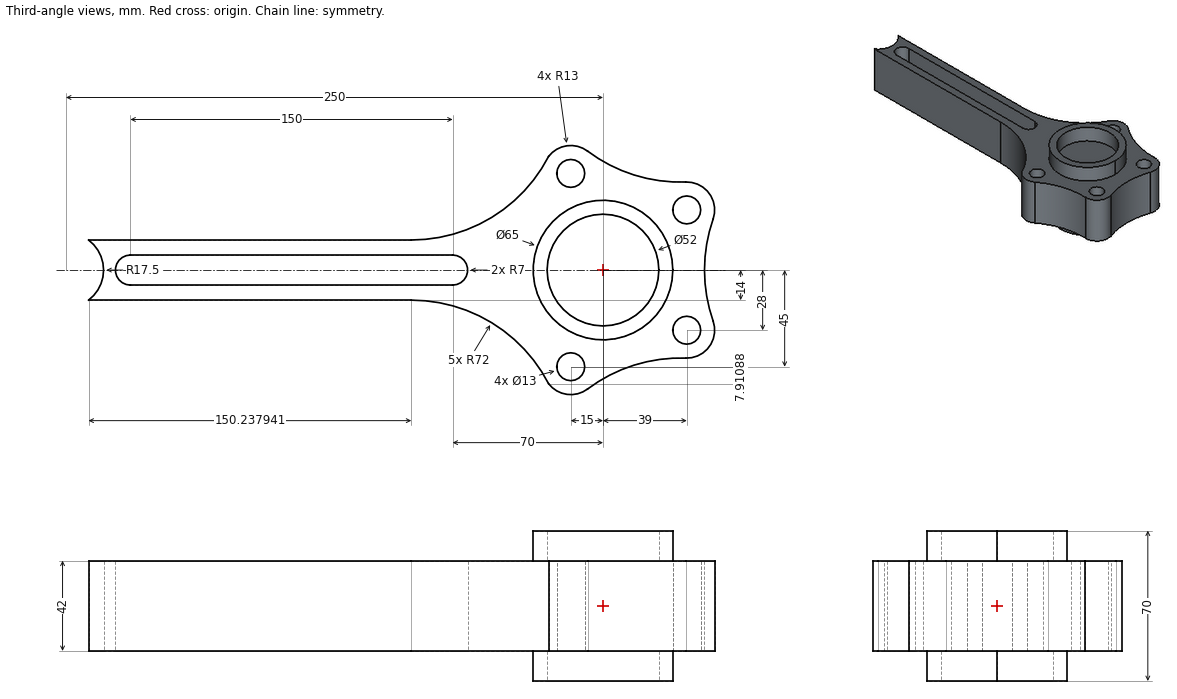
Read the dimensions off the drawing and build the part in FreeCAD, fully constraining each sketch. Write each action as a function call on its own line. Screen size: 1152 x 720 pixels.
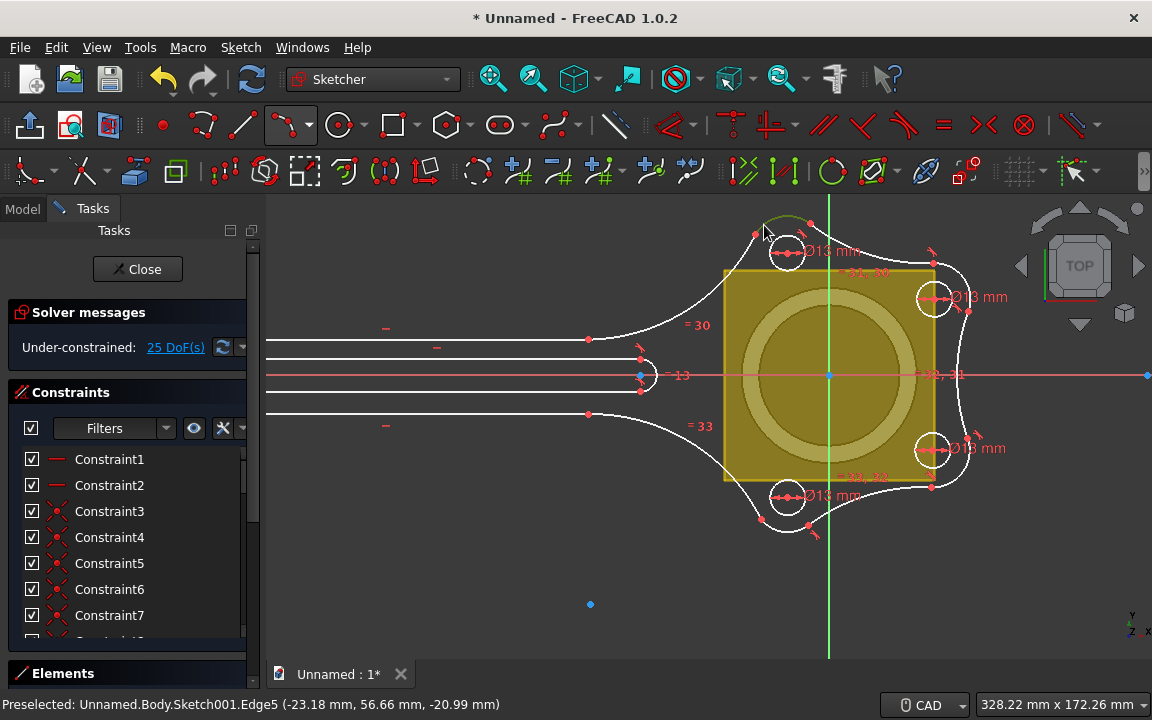
click(969, 291)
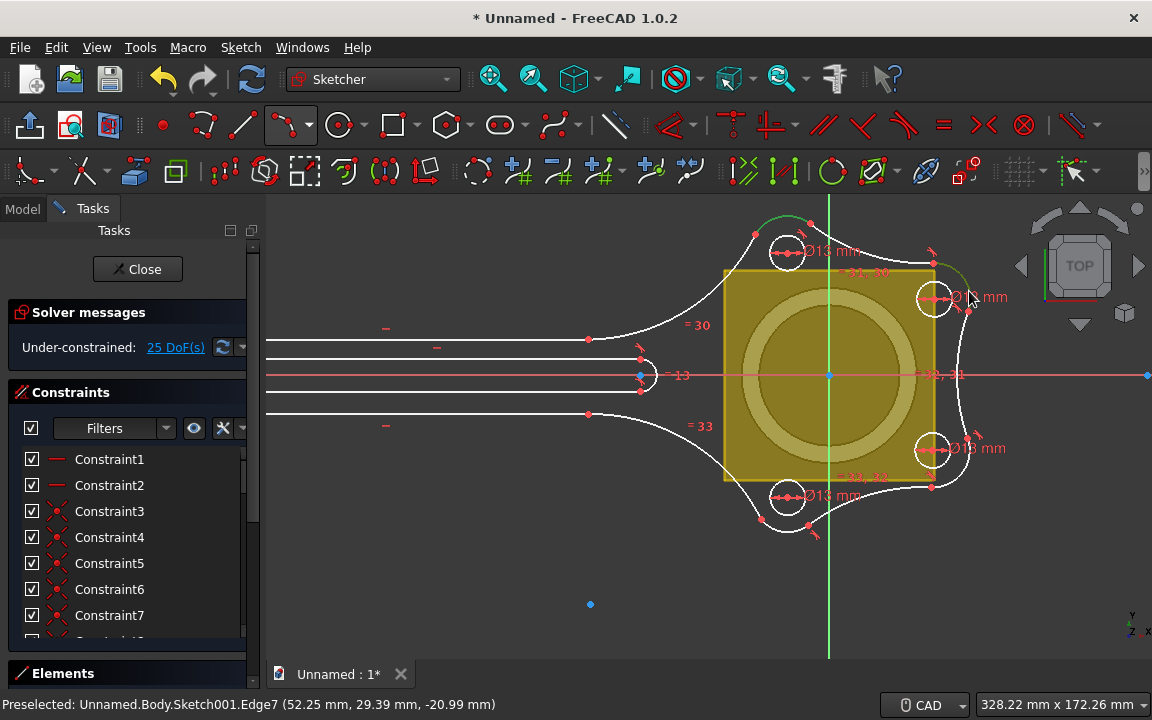
click(952, 482)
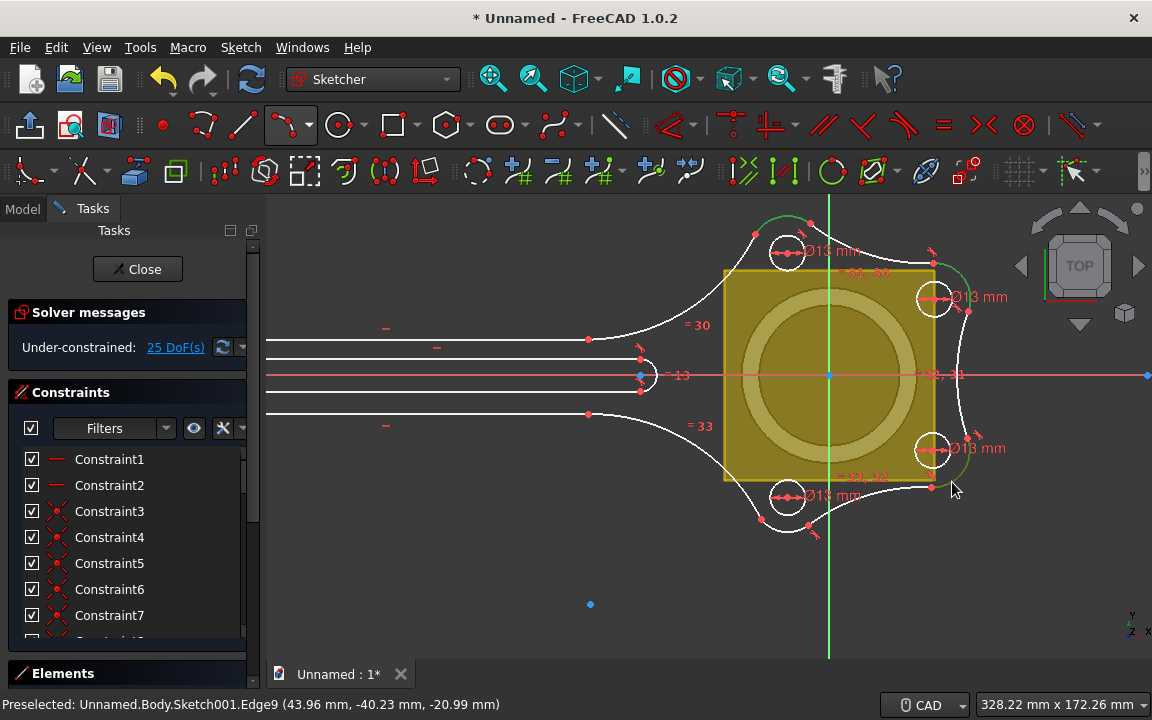
click(774, 529)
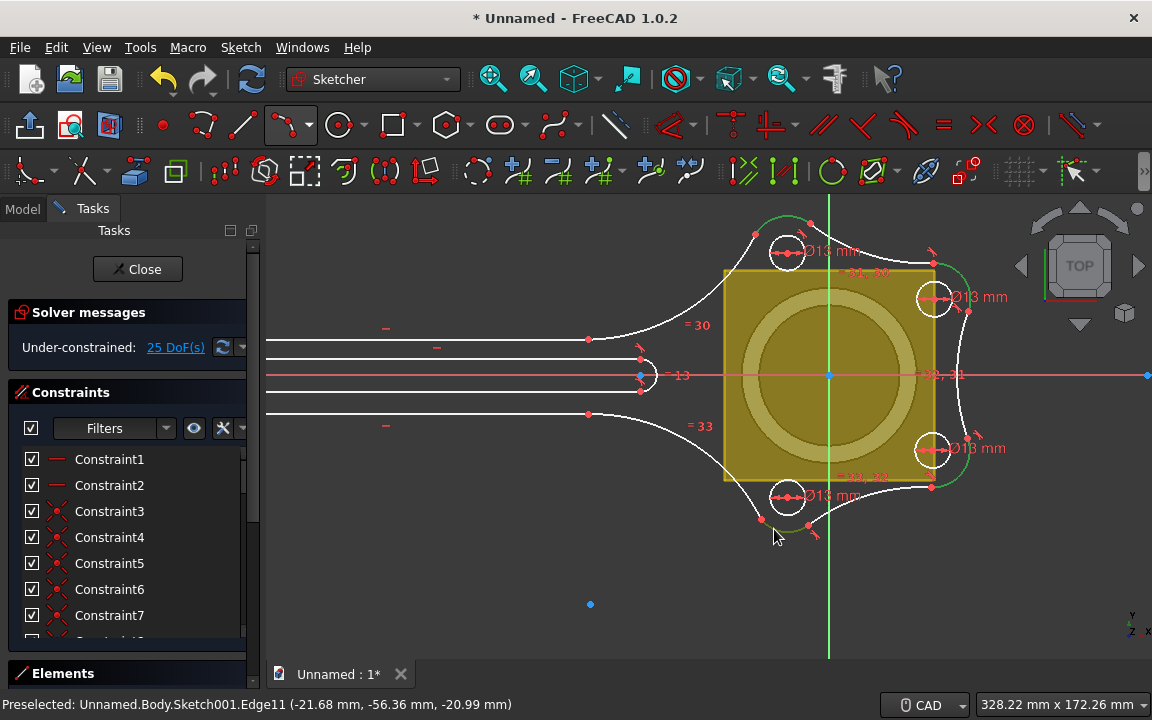
click(944, 126)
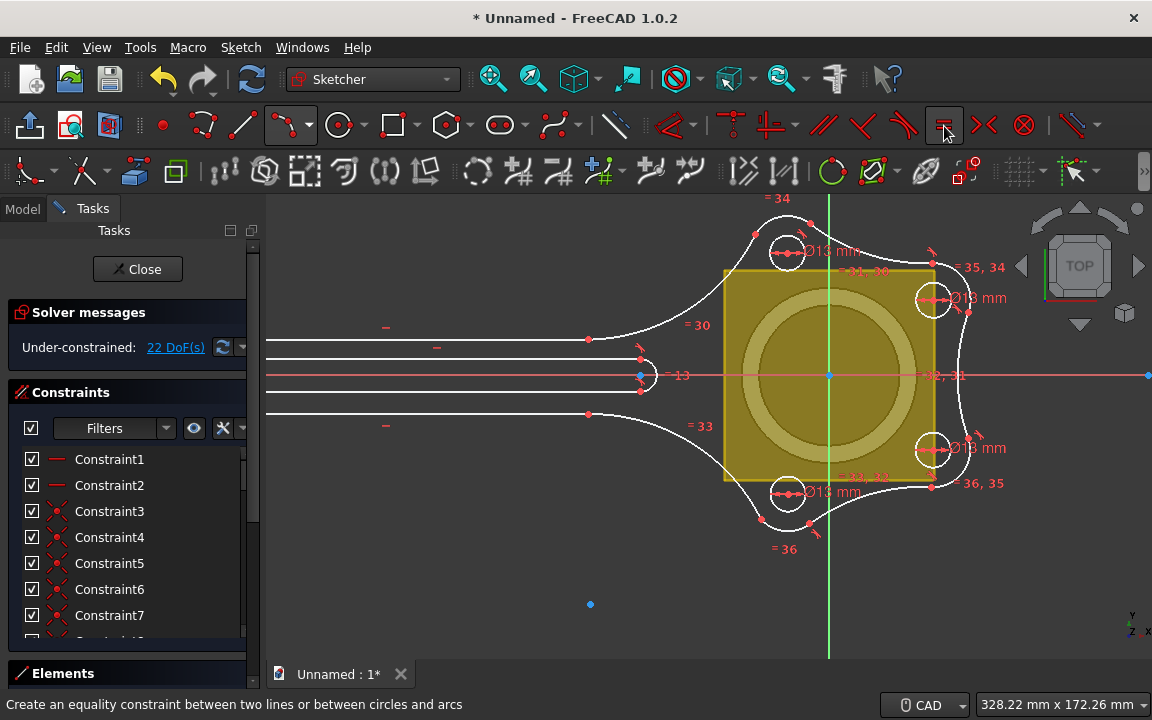
scroll(773, 530, down, 2)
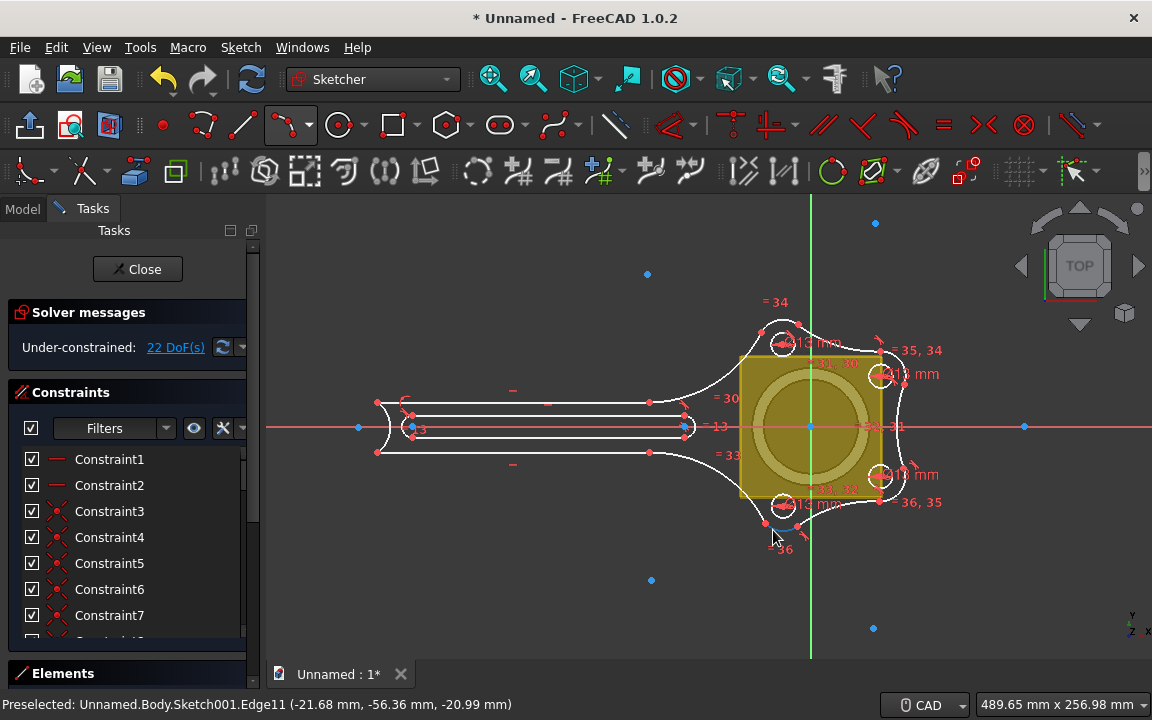
click(359, 428)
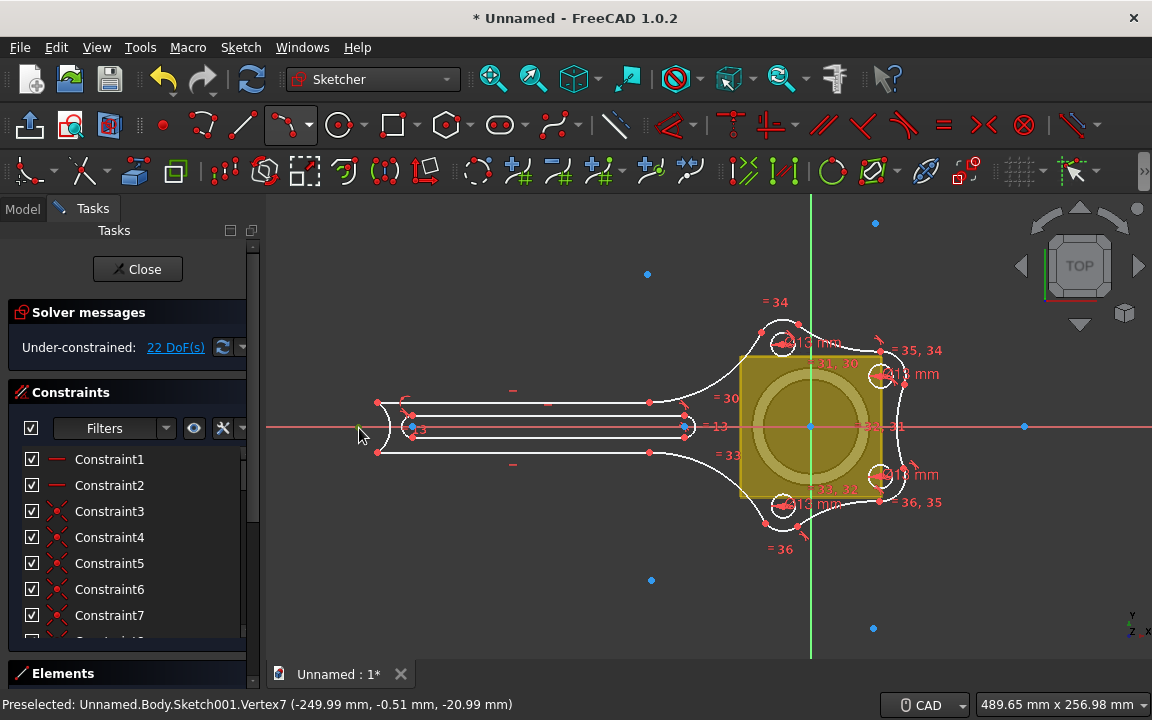
click(344, 427)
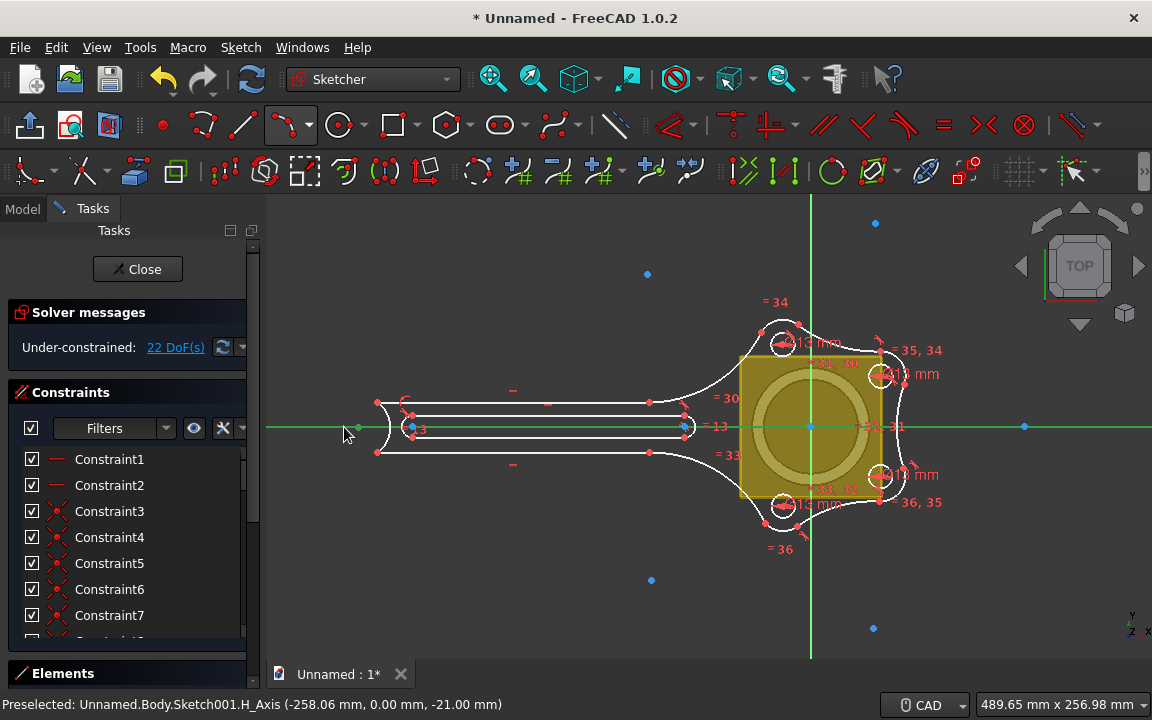
click(732, 126)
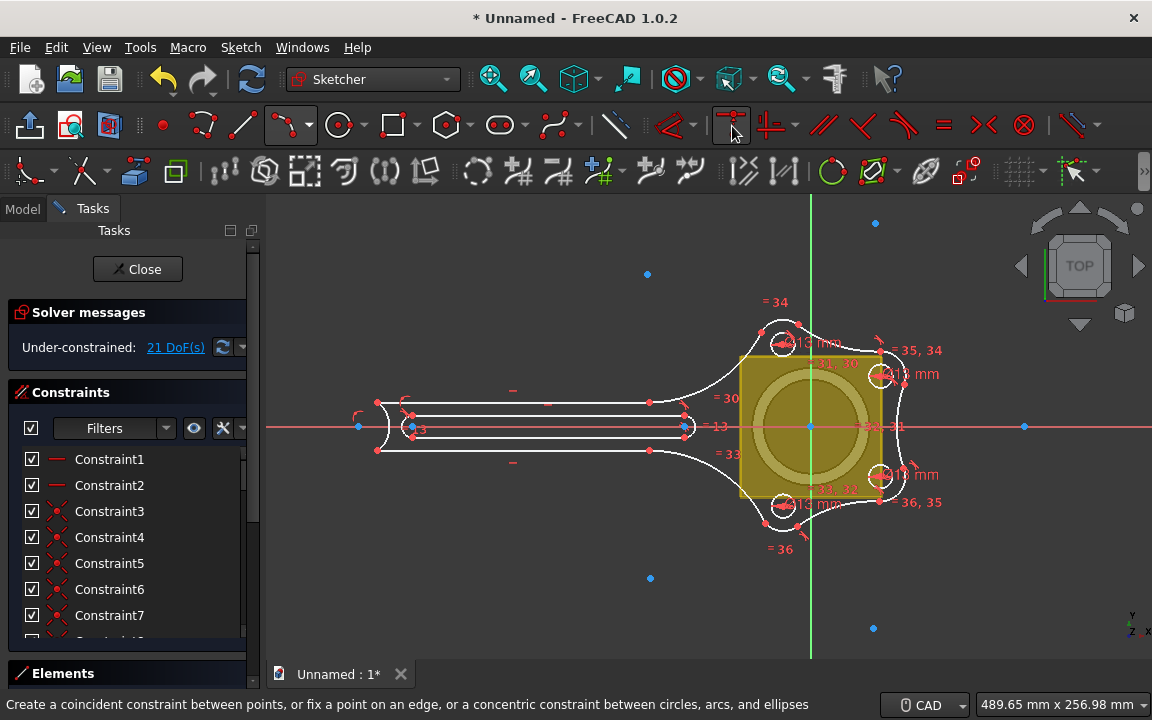
scroll(367, 426, down, 1)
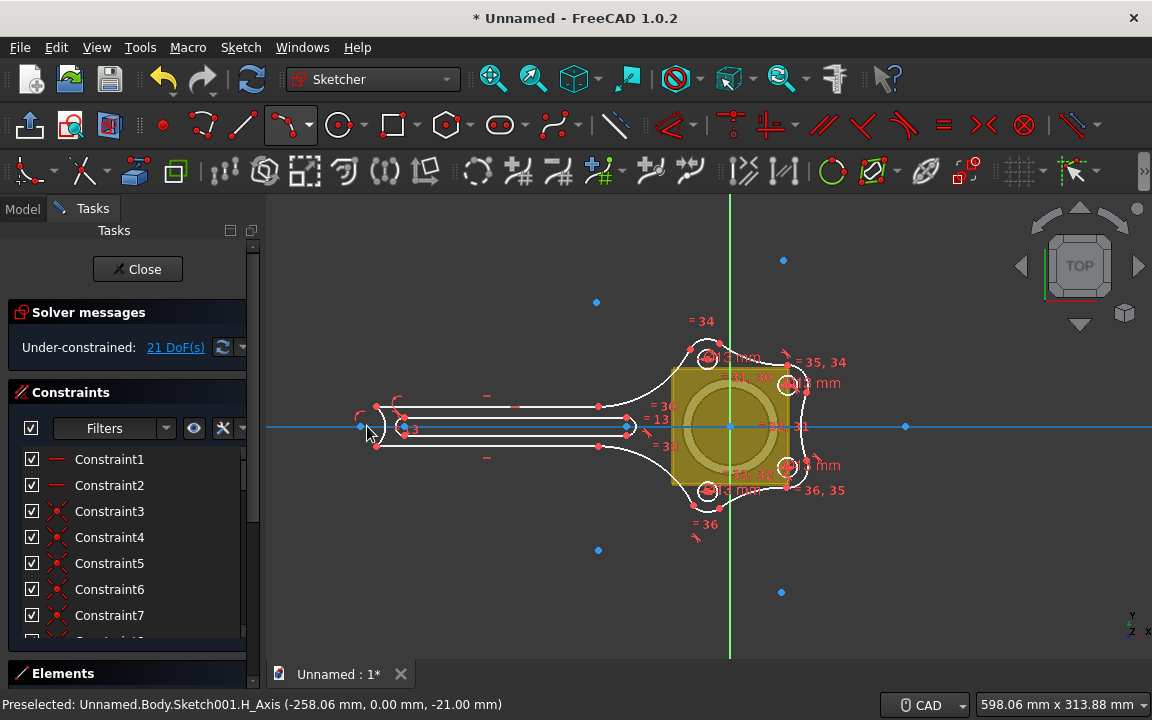
click(905, 427)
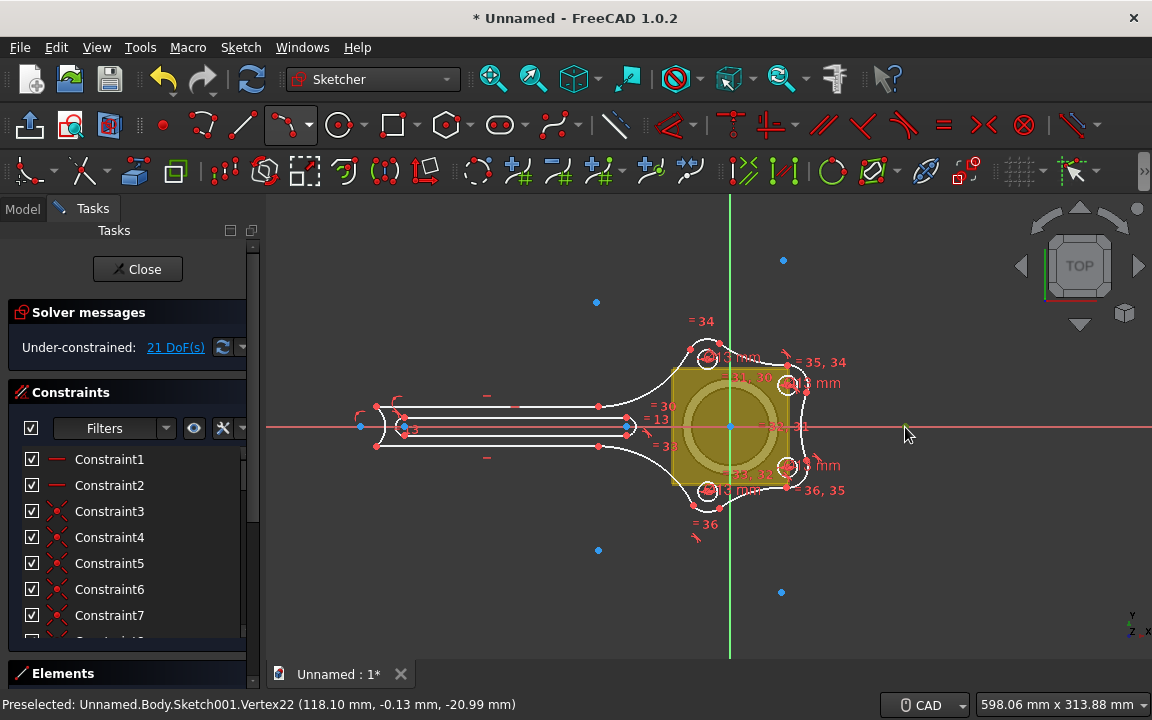
click(343, 427)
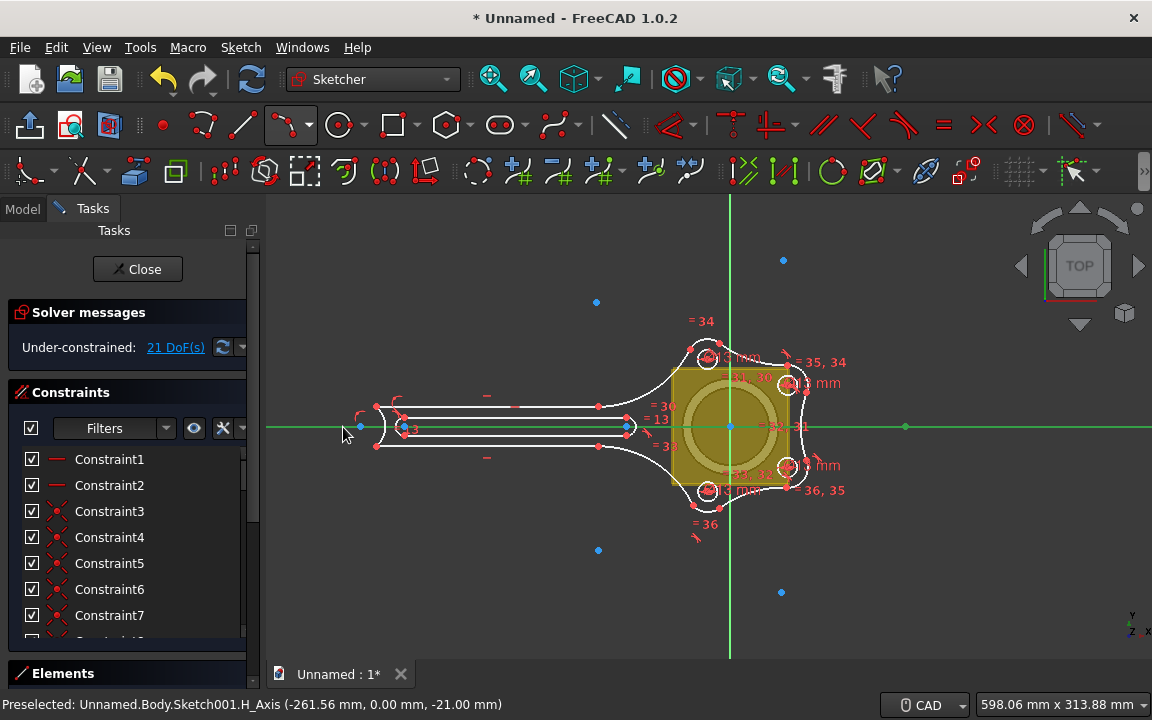
click(732, 126)